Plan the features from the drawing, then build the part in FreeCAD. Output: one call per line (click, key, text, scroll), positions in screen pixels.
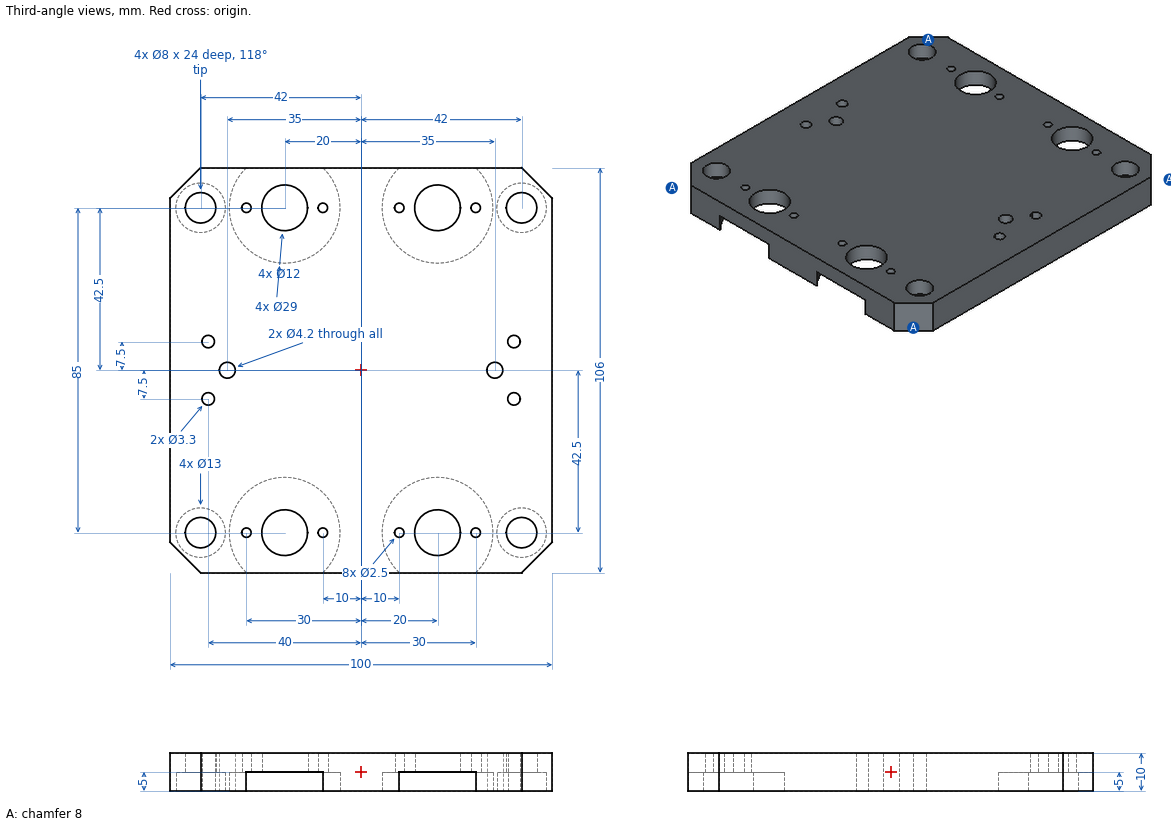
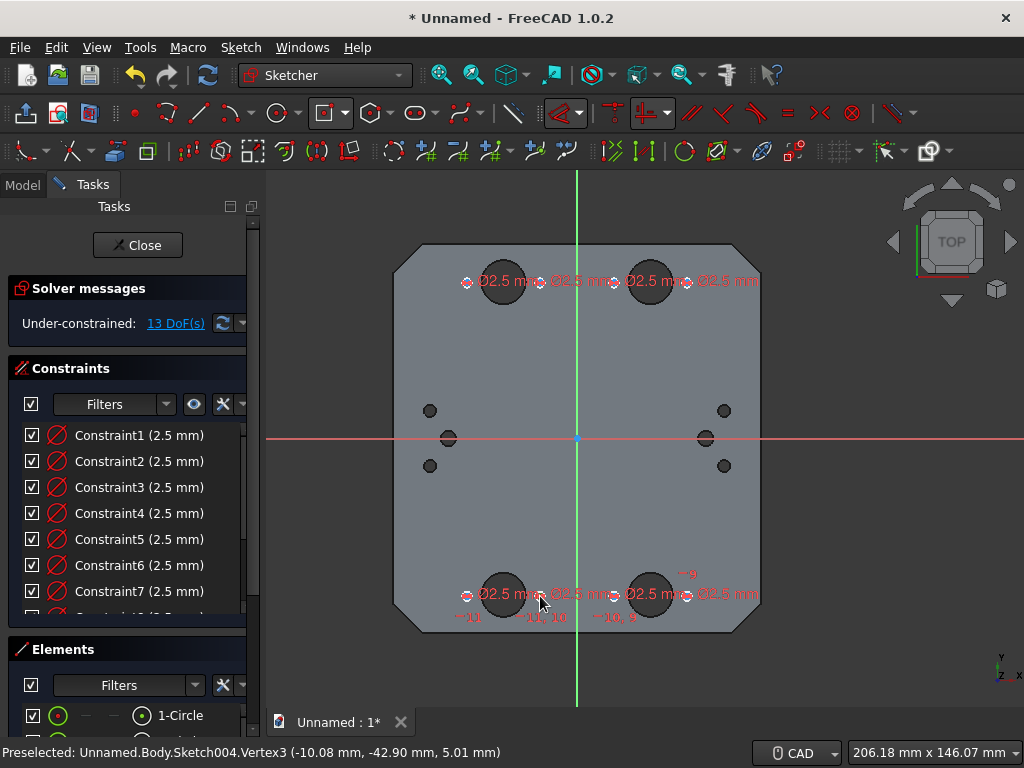
click(540, 283)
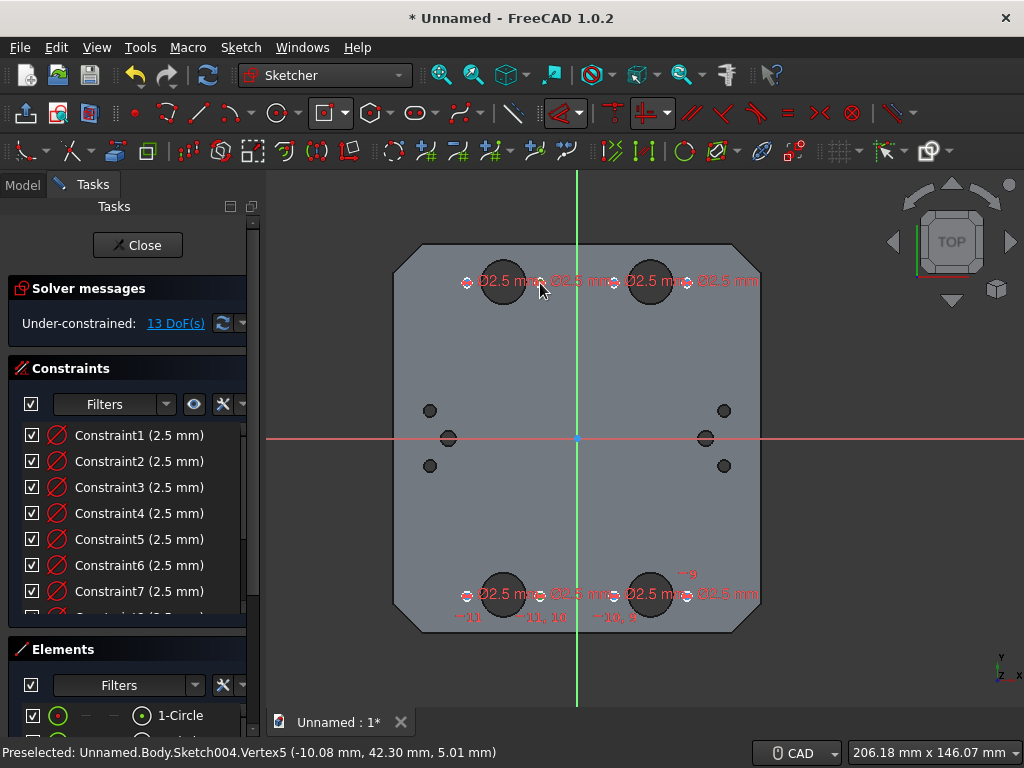
click(670, 114)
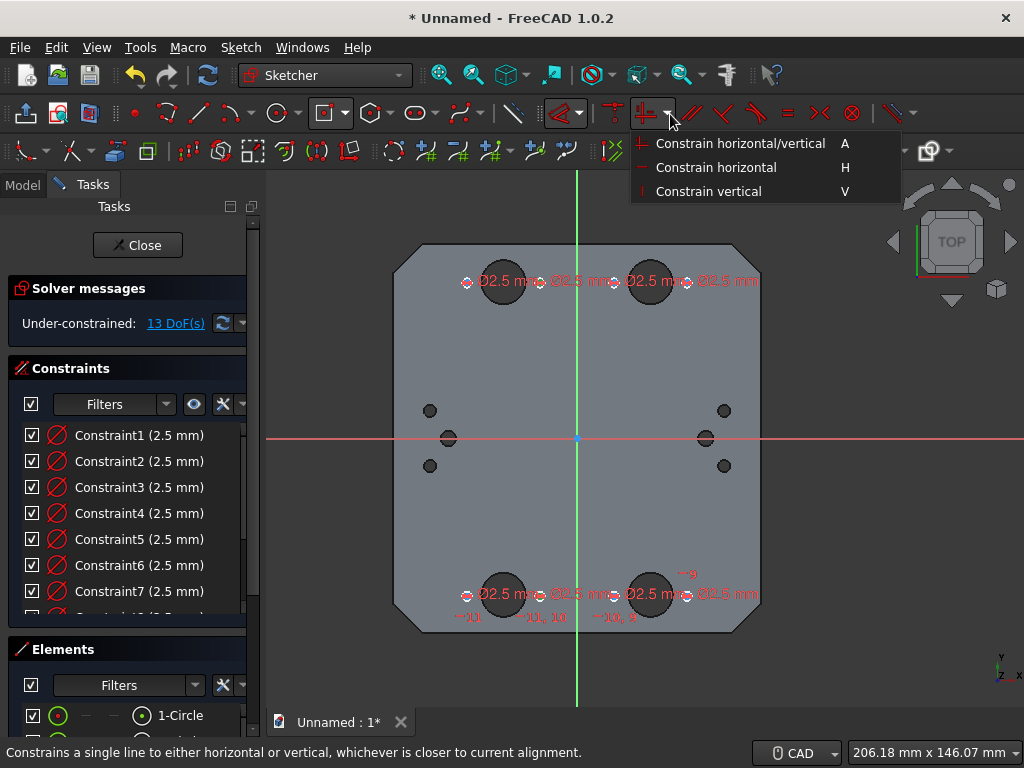
click(766, 191)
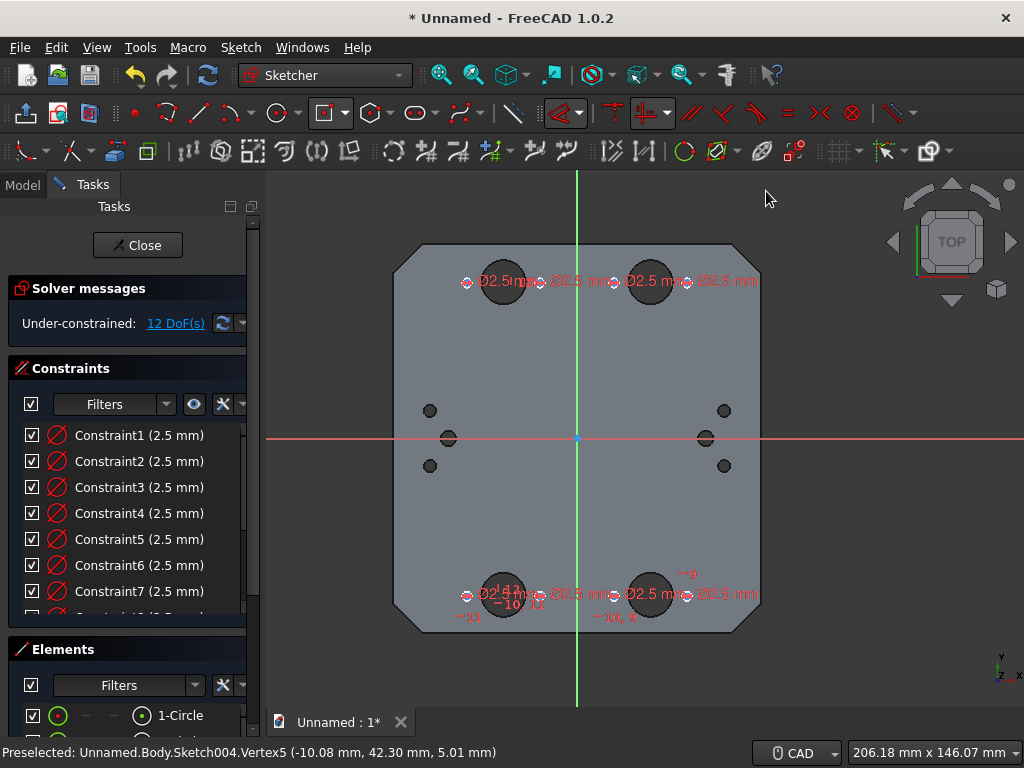
click(467, 596)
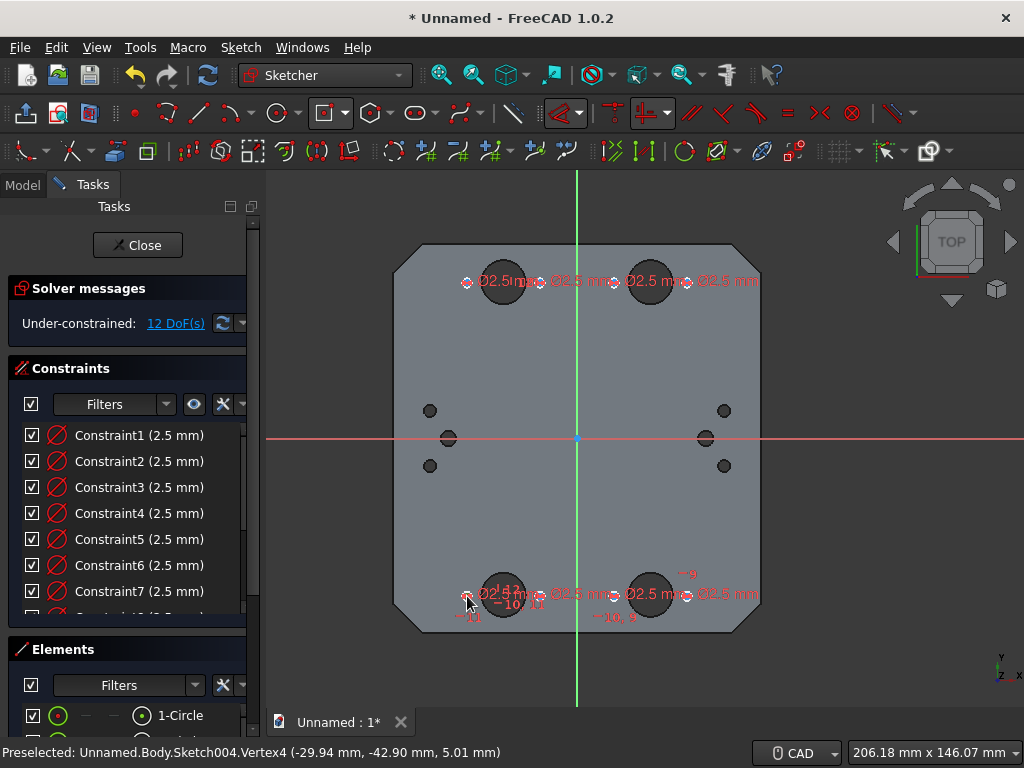
click(467, 283)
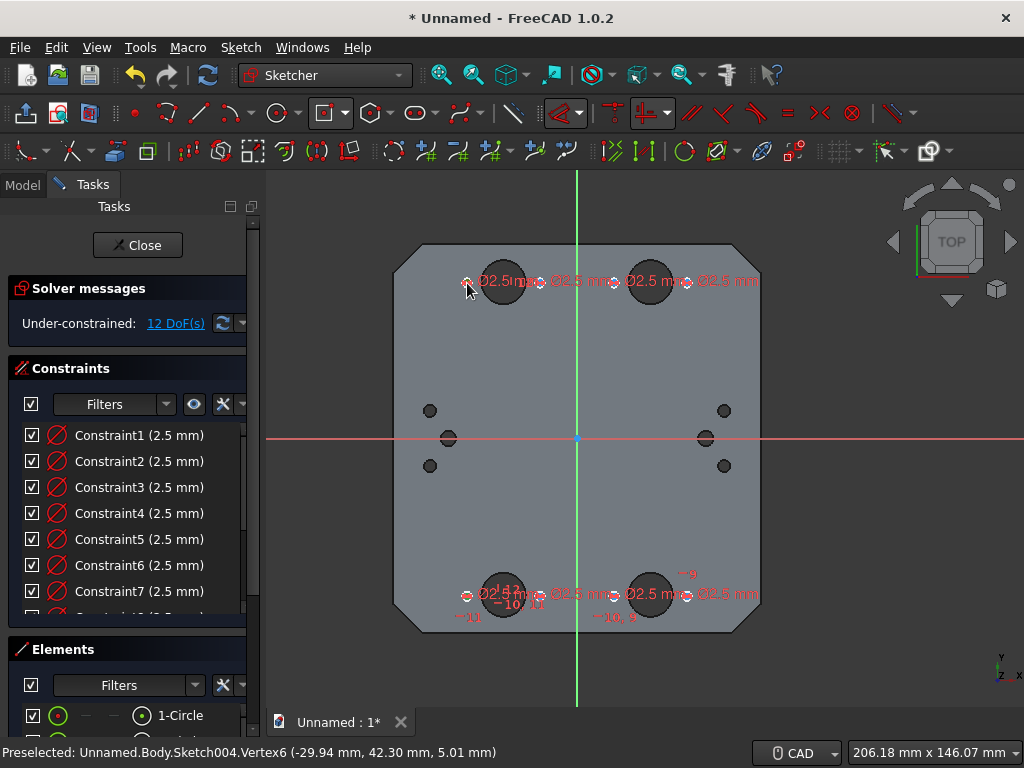
click(670, 114)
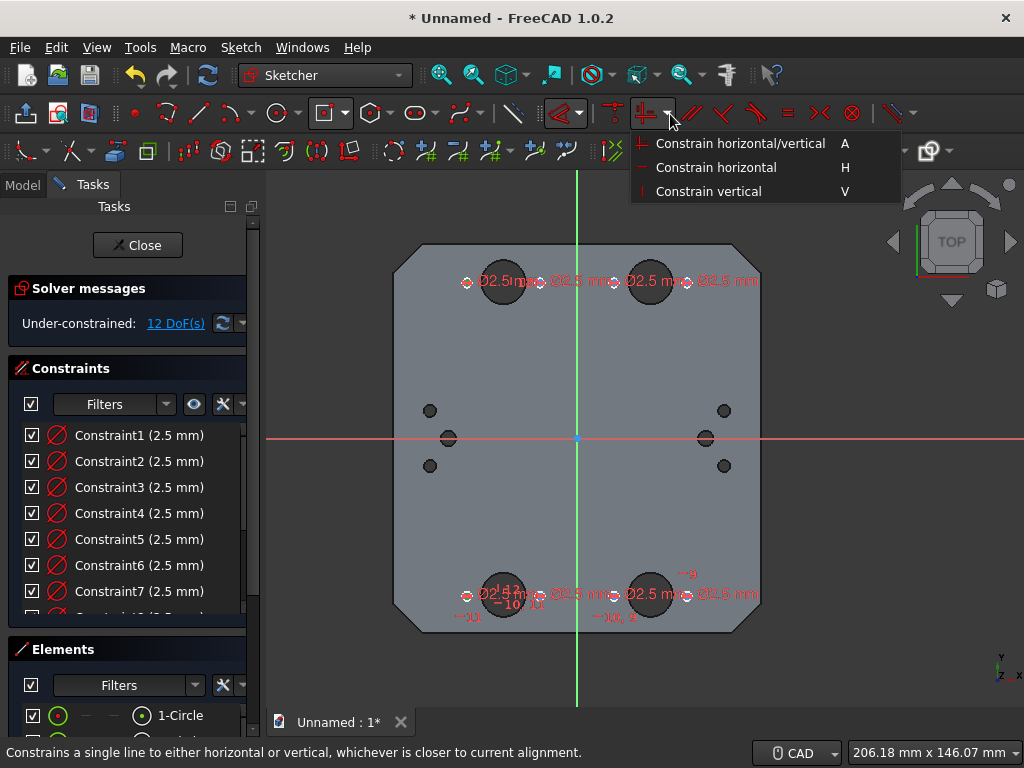
click(766, 191)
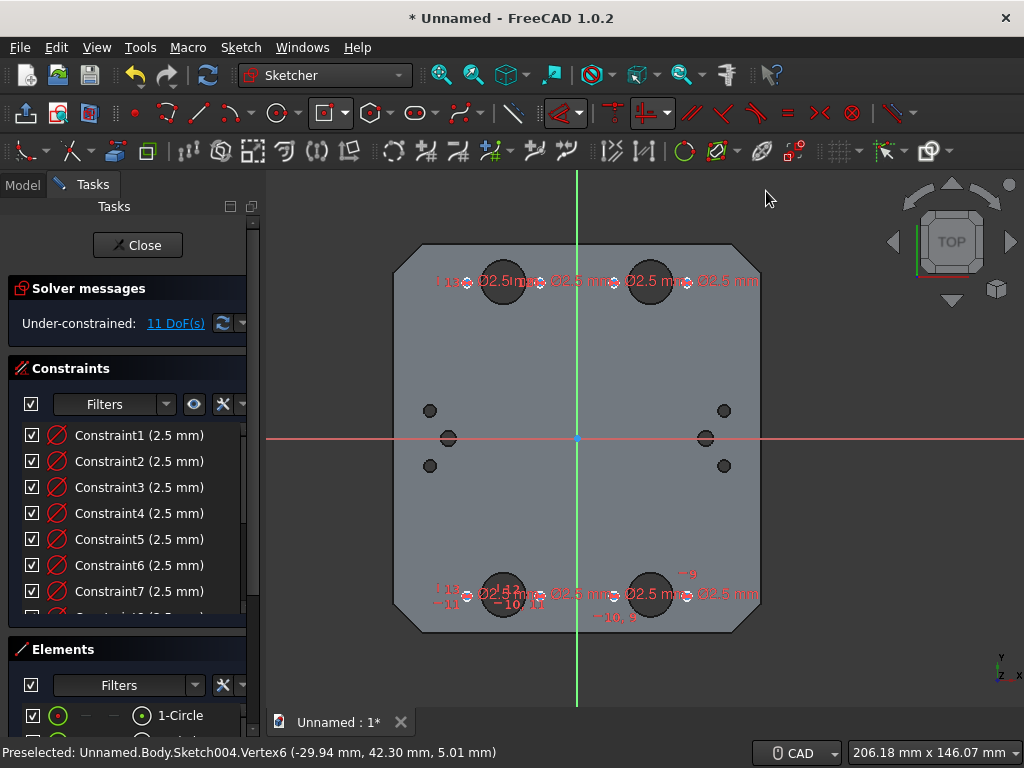
click(540, 283)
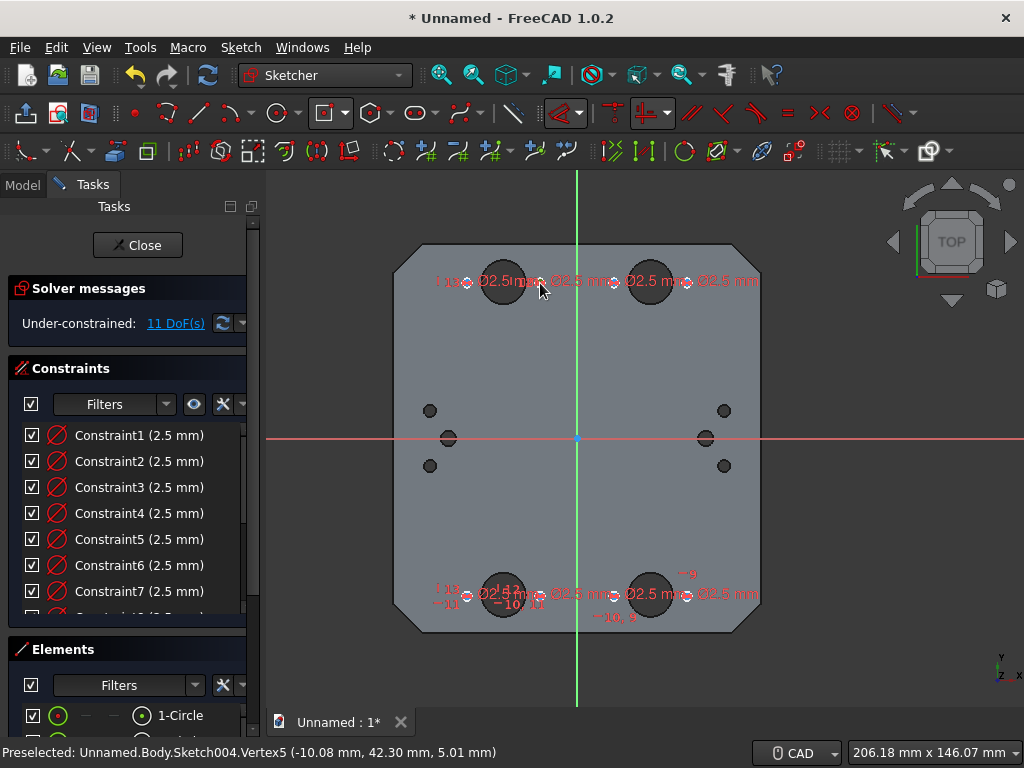
click(467, 283)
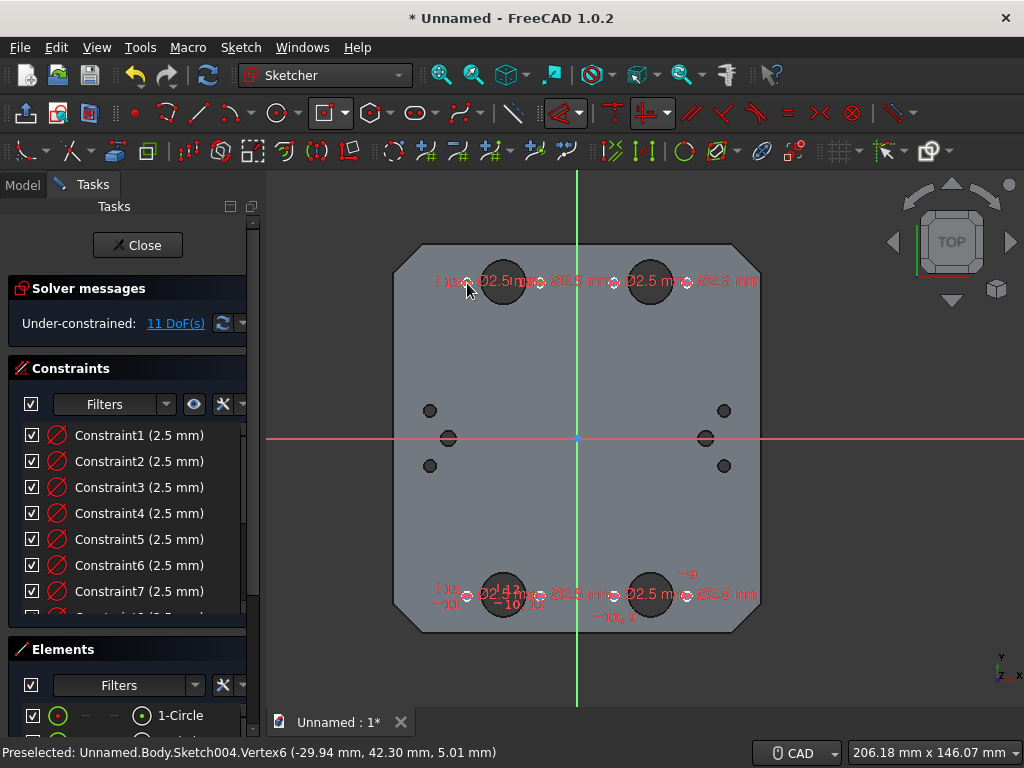
key(h)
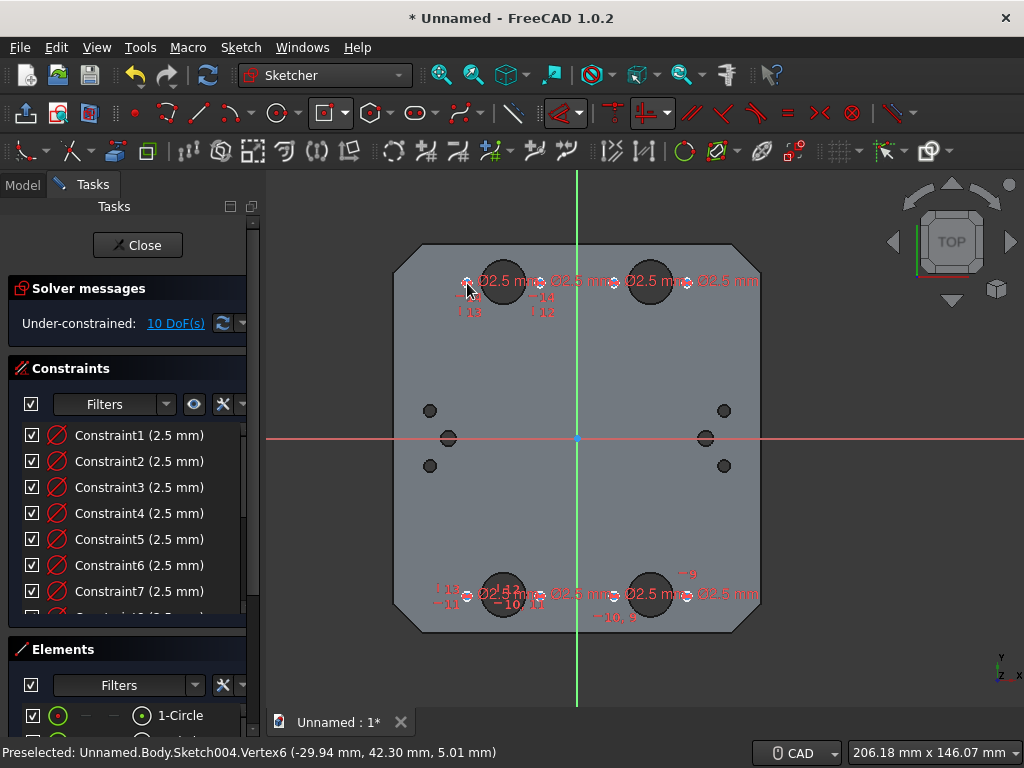
click(614, 596)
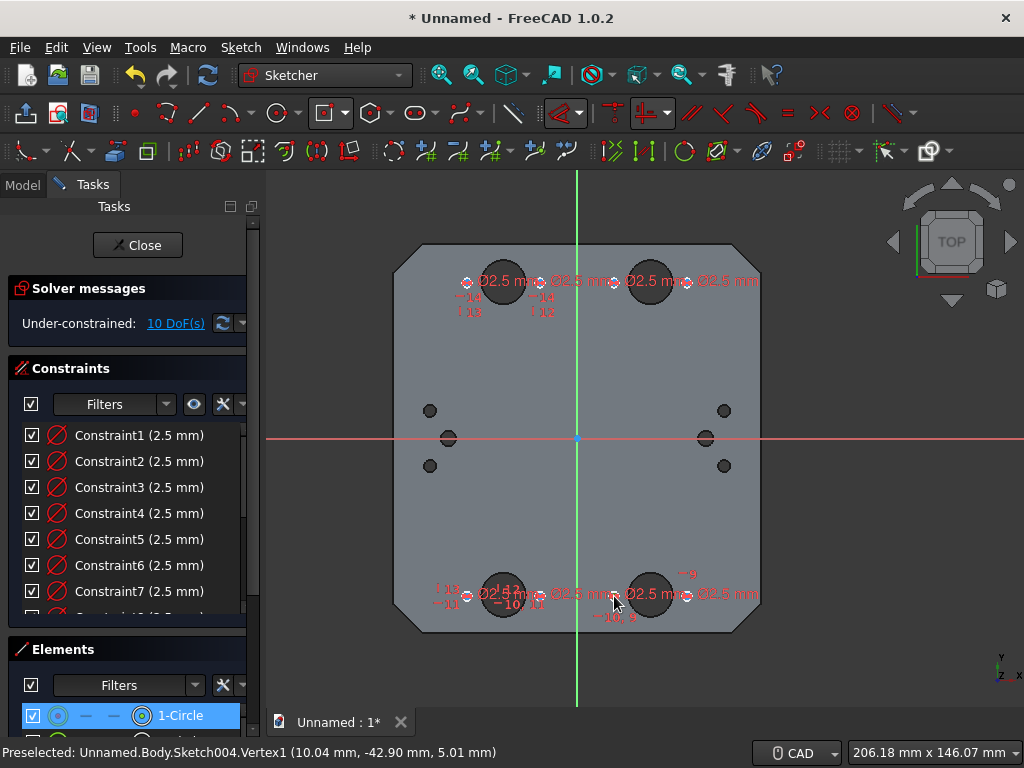
click(614, 283)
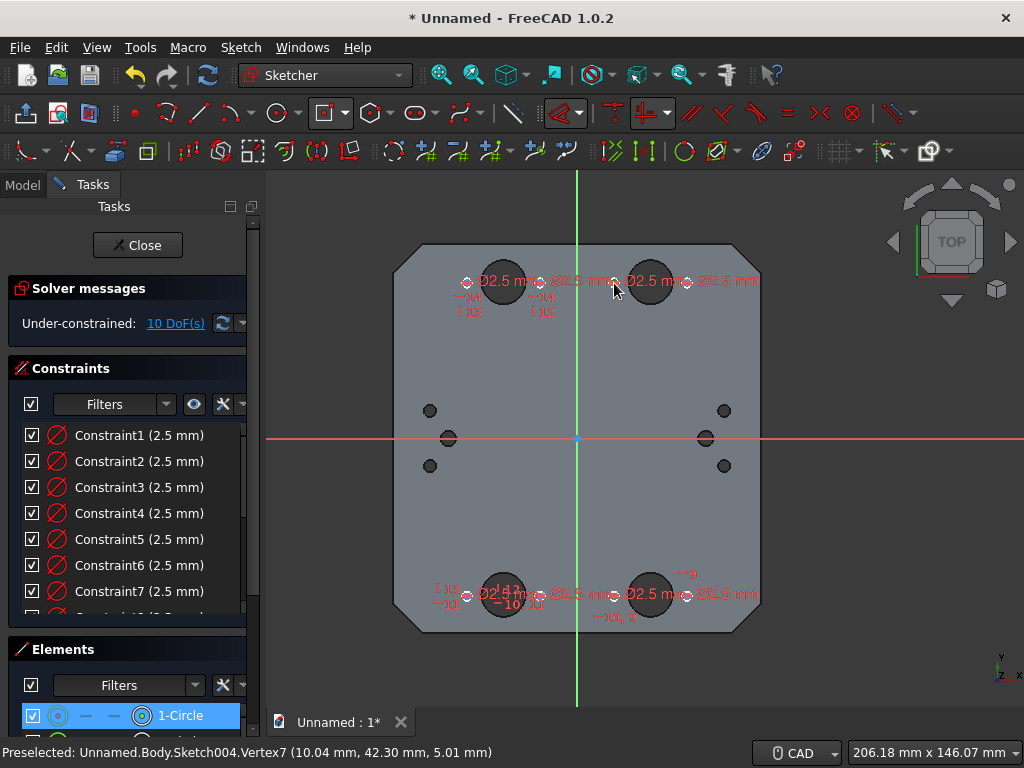
click(670, 114)